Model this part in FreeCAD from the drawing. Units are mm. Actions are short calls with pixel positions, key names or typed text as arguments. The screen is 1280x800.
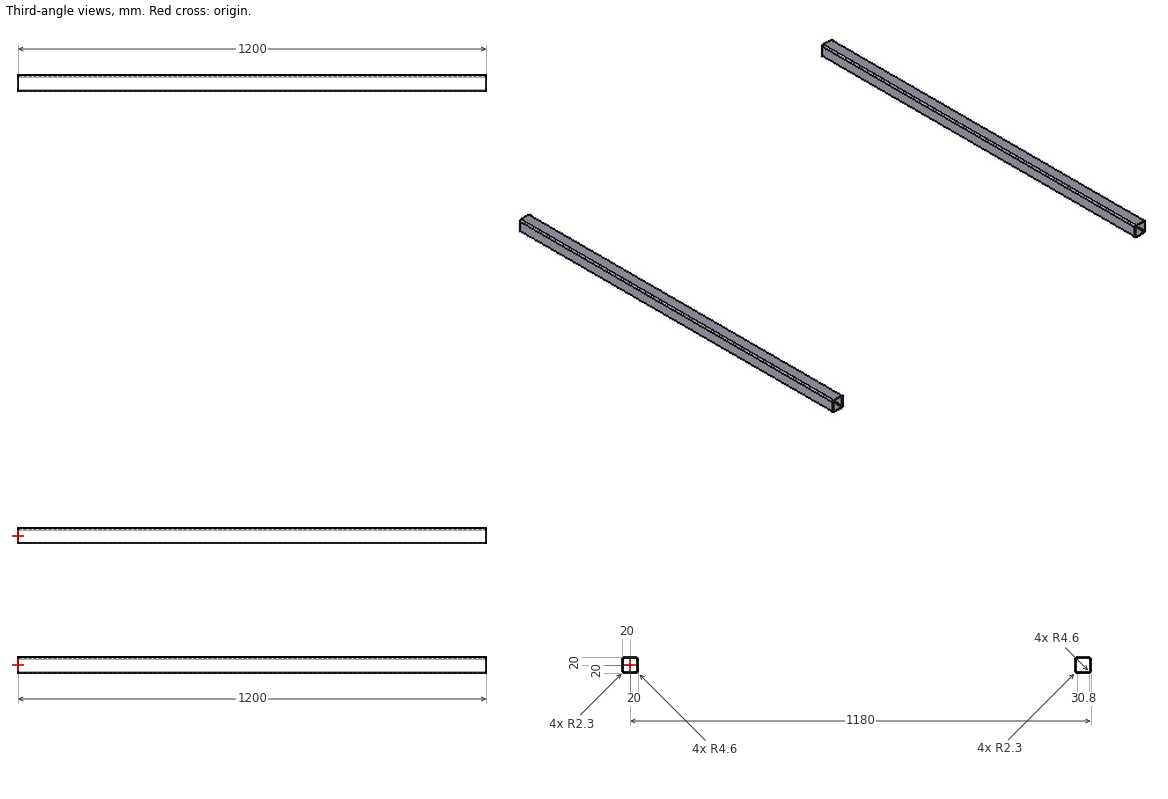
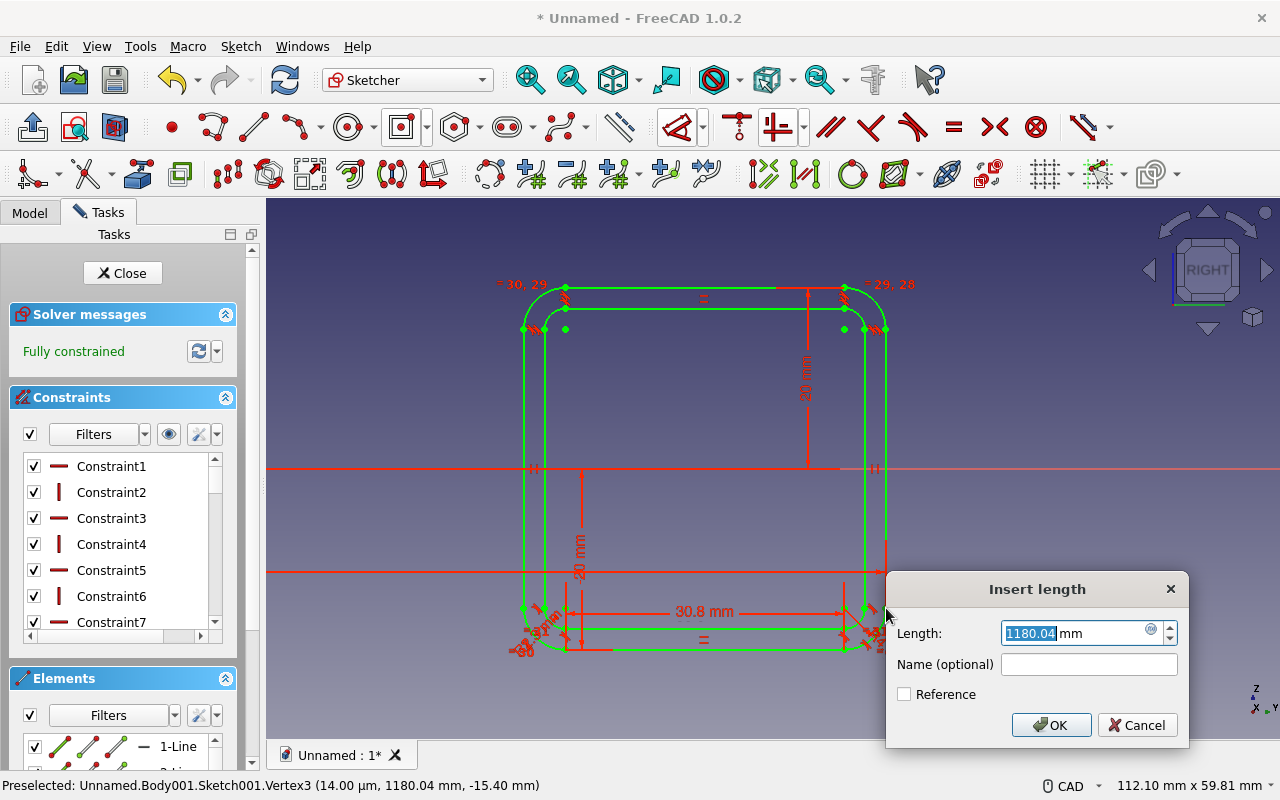
text(1180)
key(Return)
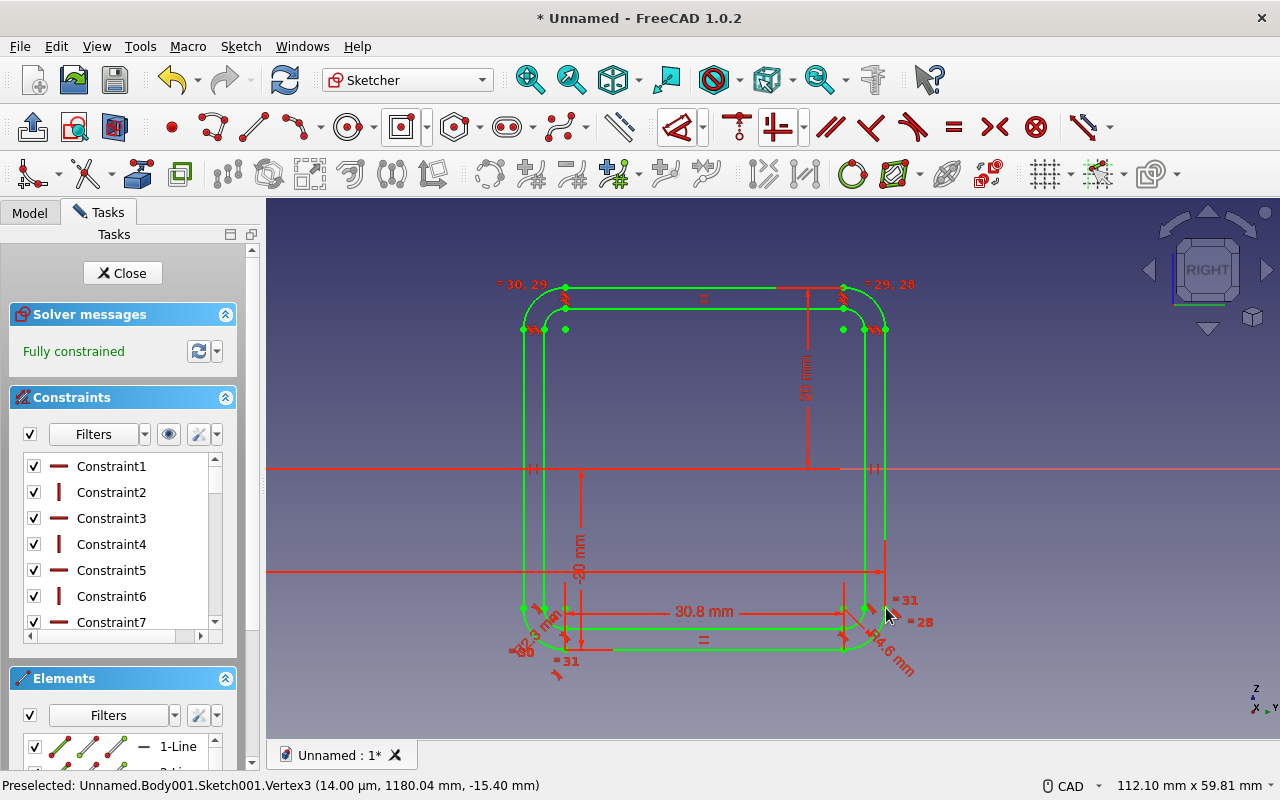
click(123, 273)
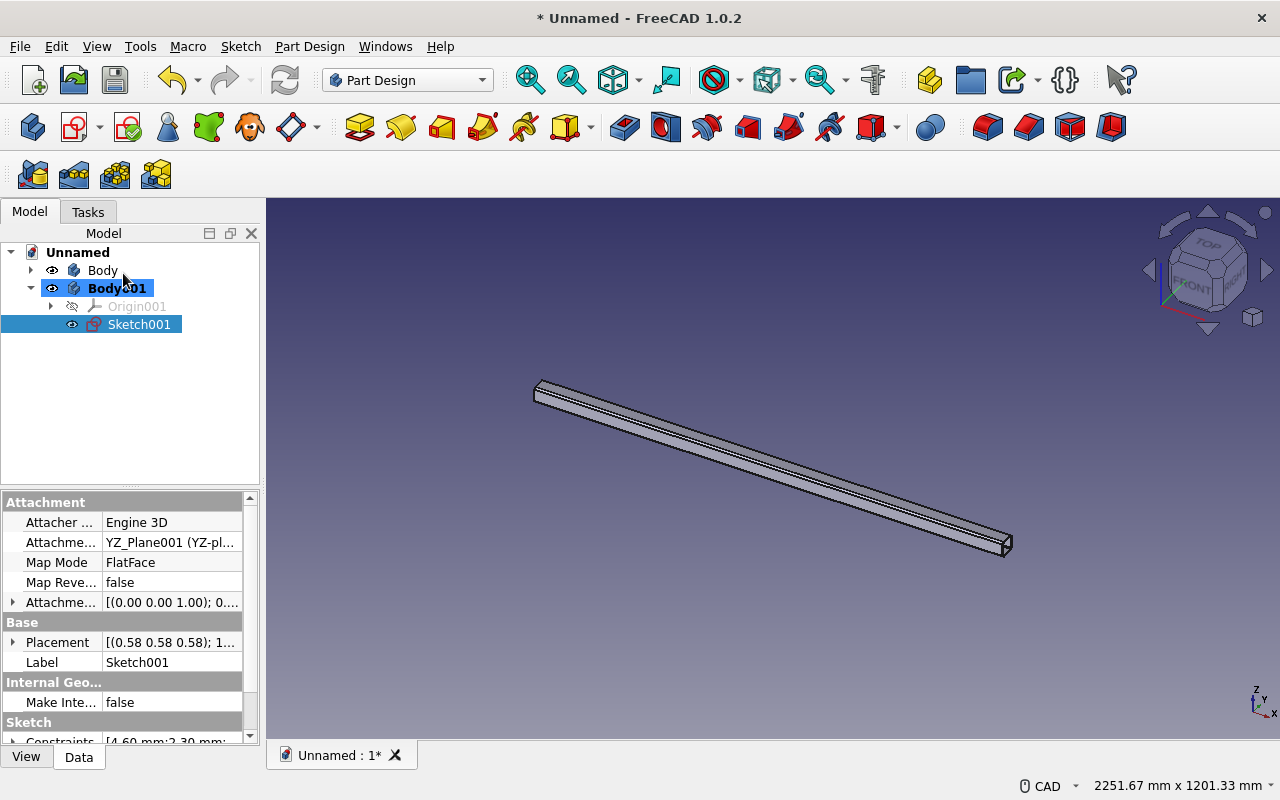
click(360, 128)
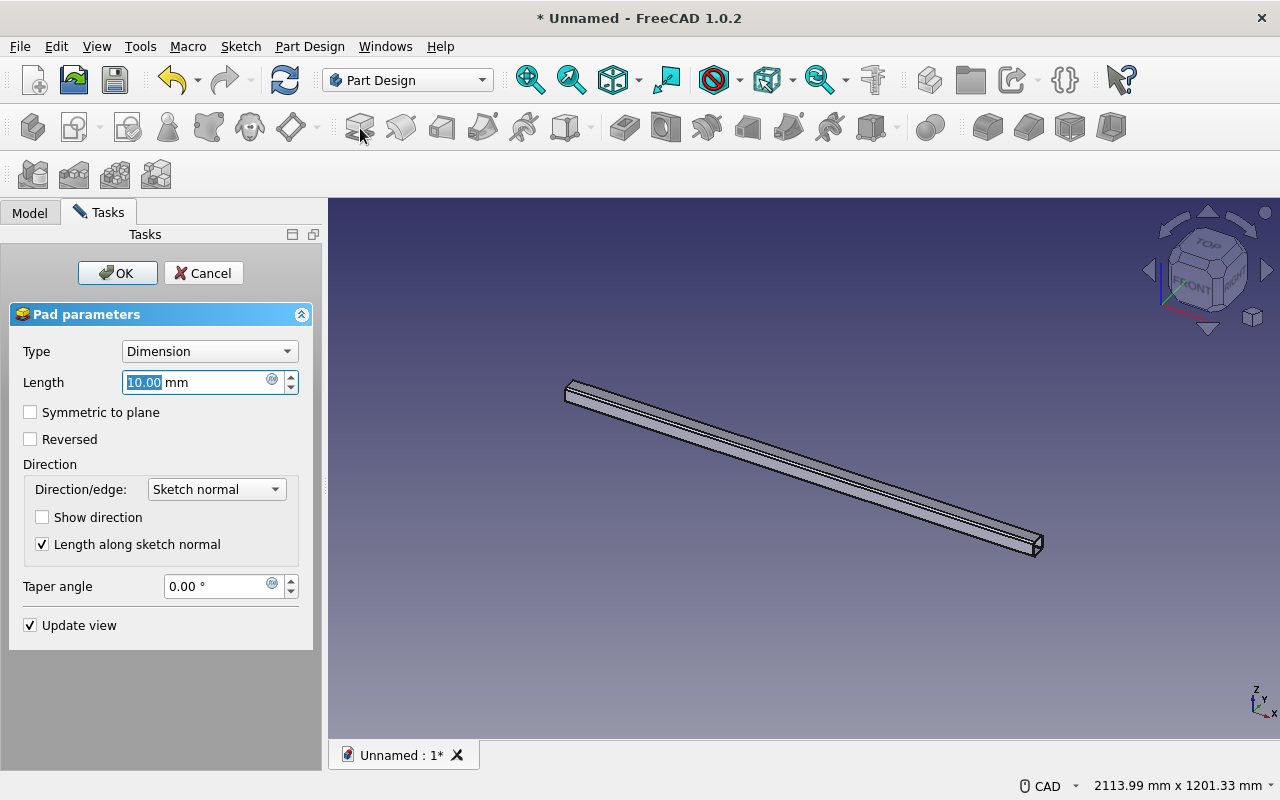
text(1200)
key(Tab)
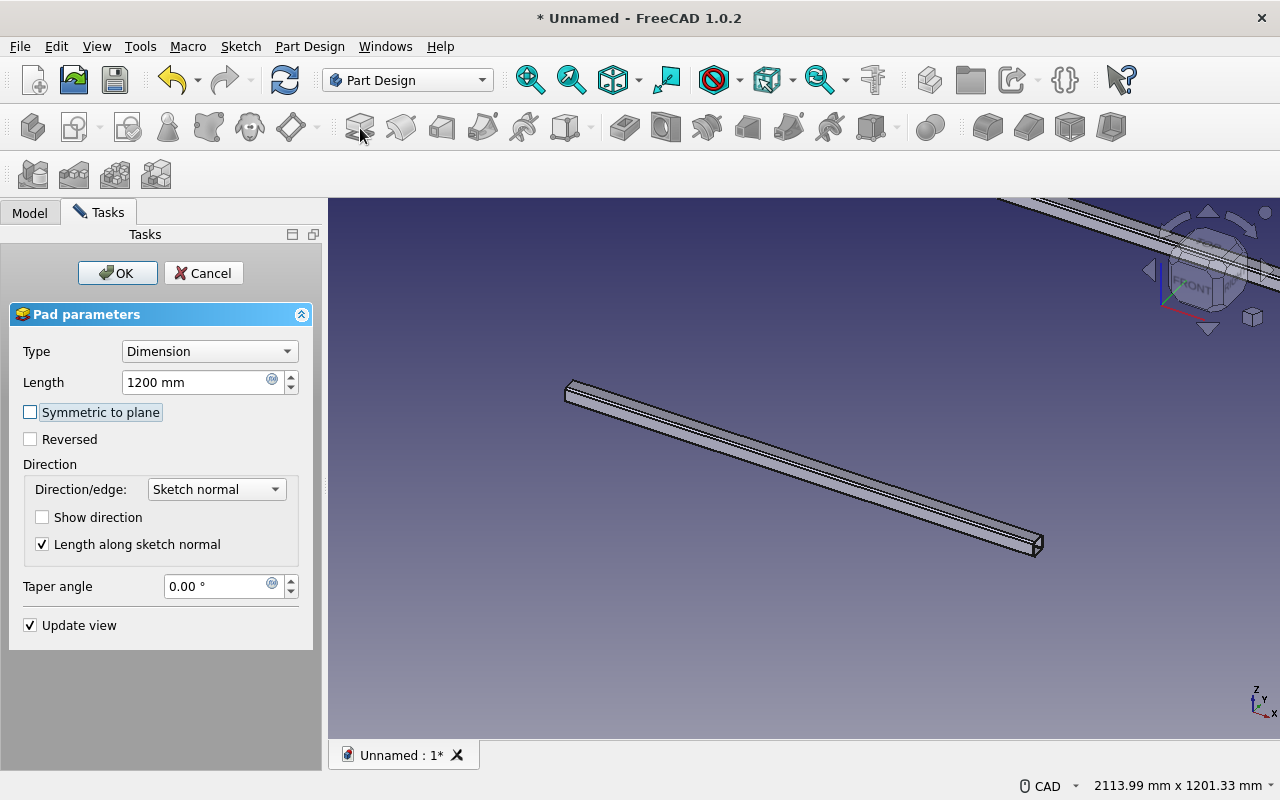
click(118, 273)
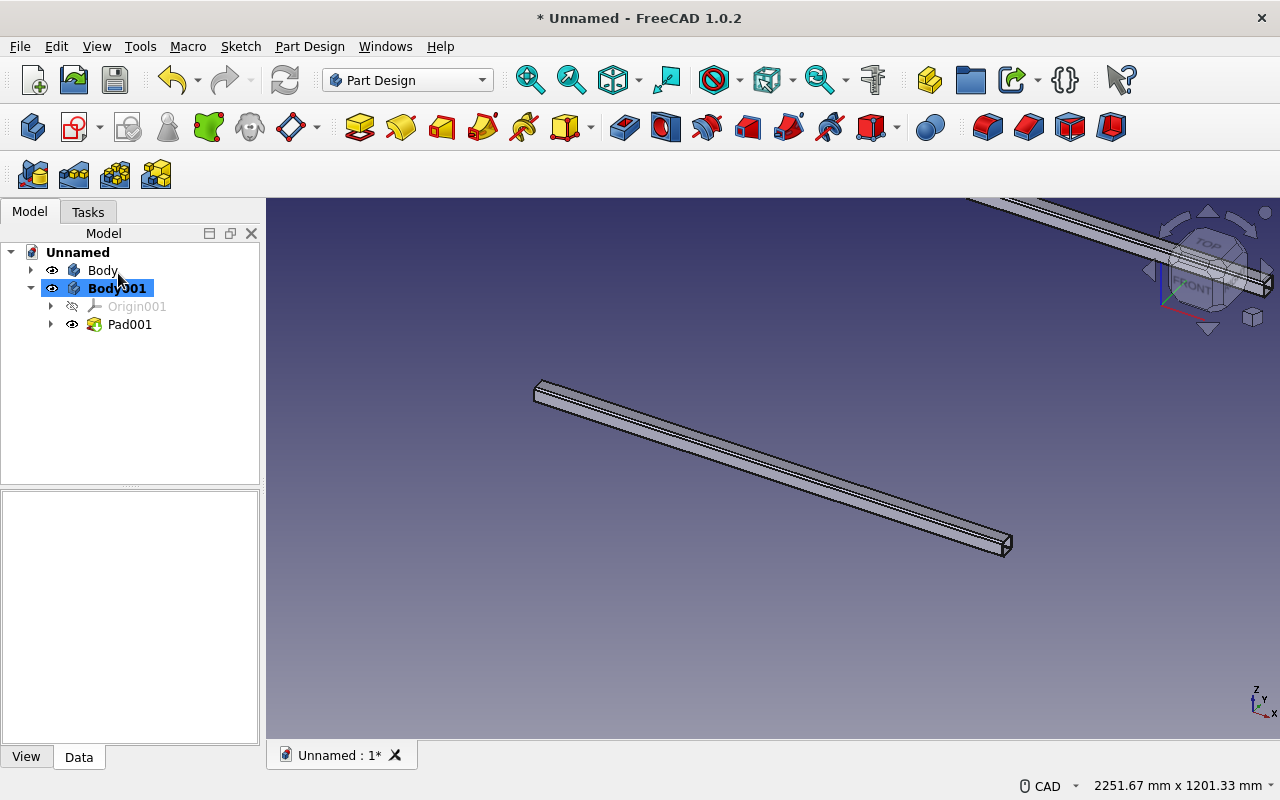
key(0)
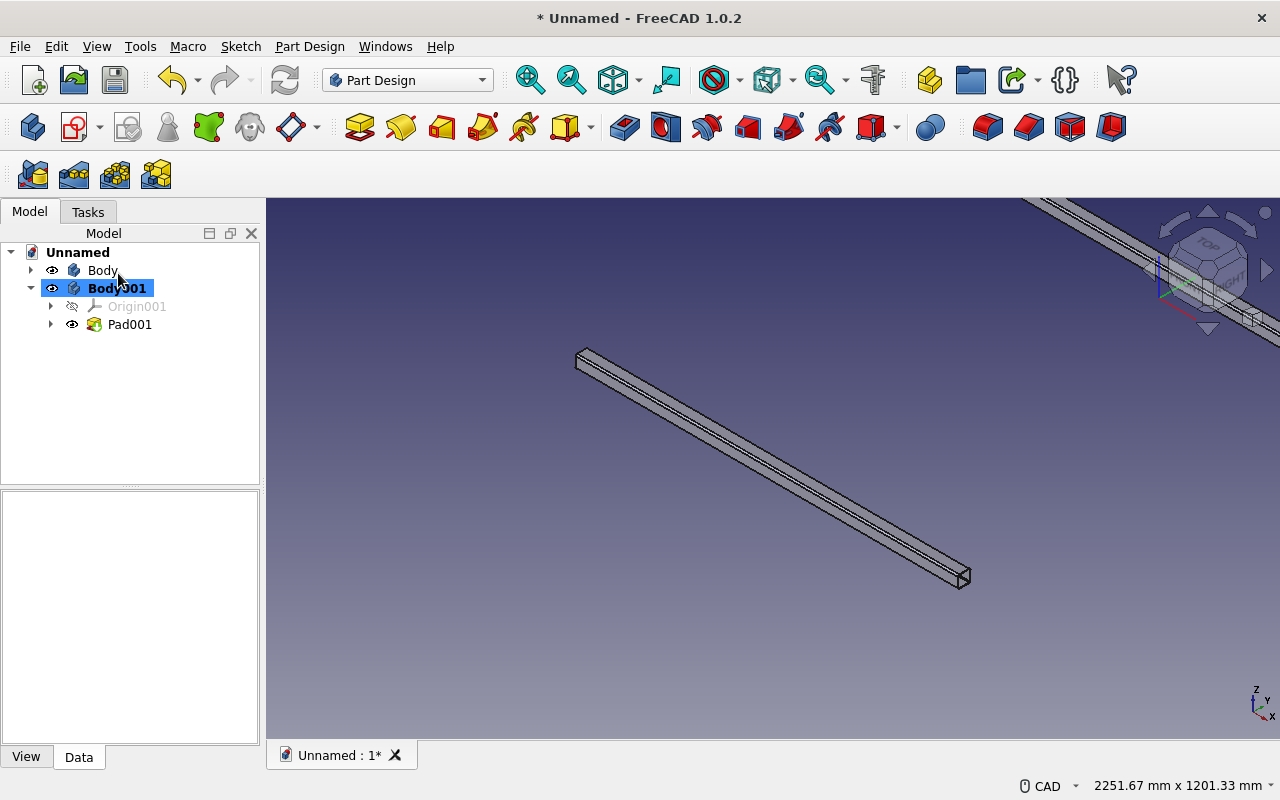
click(531, 80)